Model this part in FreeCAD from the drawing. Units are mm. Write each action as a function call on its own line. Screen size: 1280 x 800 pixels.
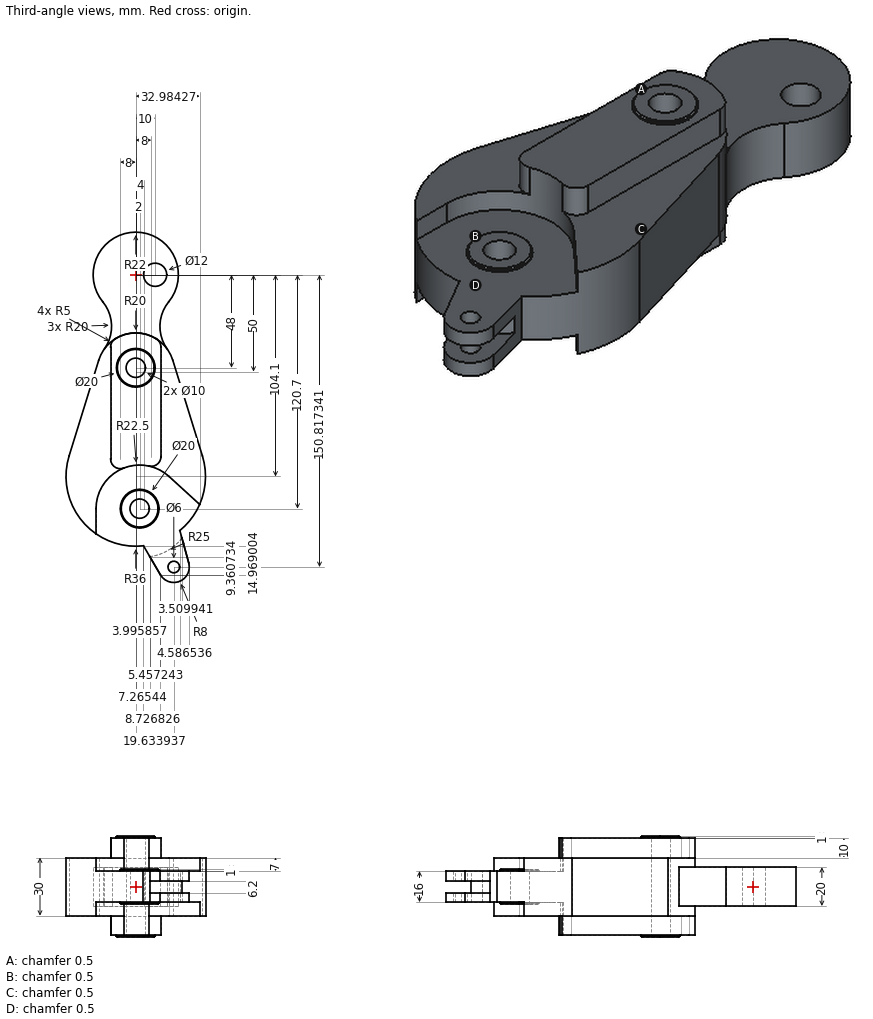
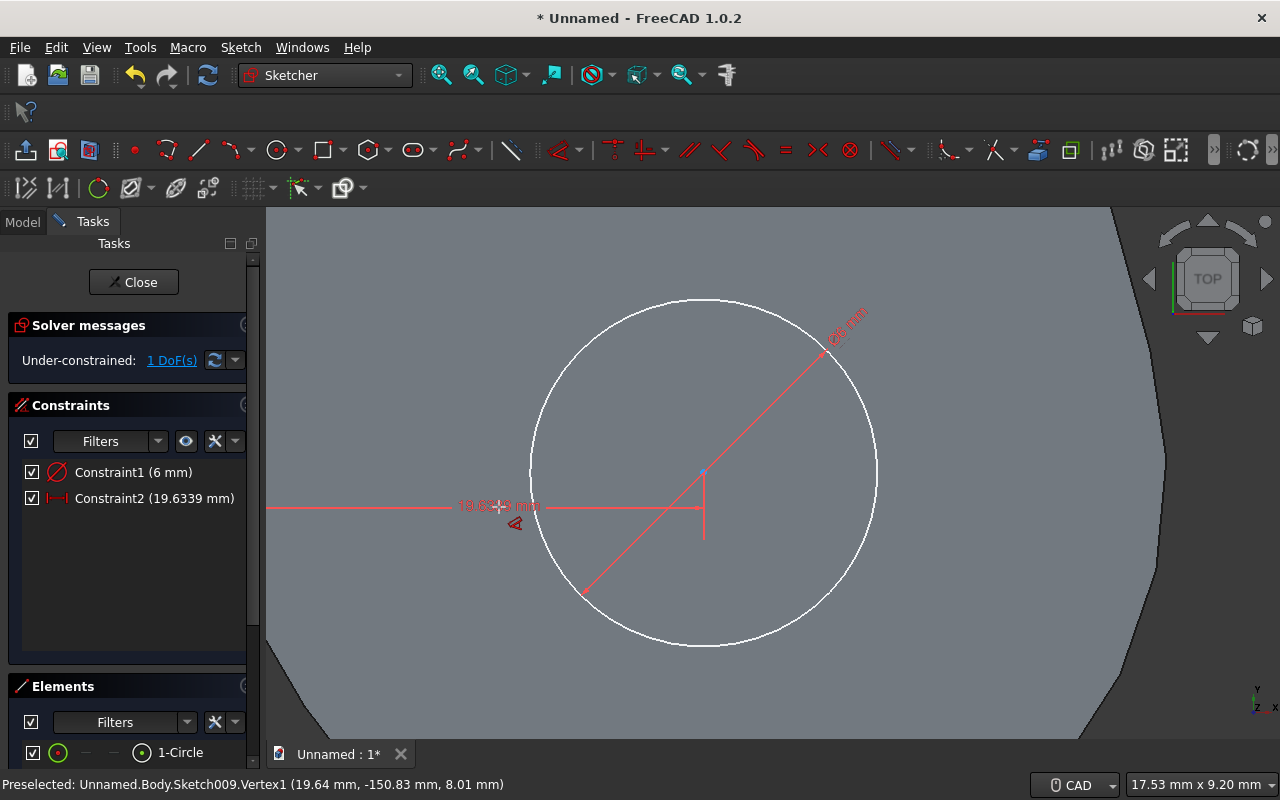
click(704, 473)
click(738, 354)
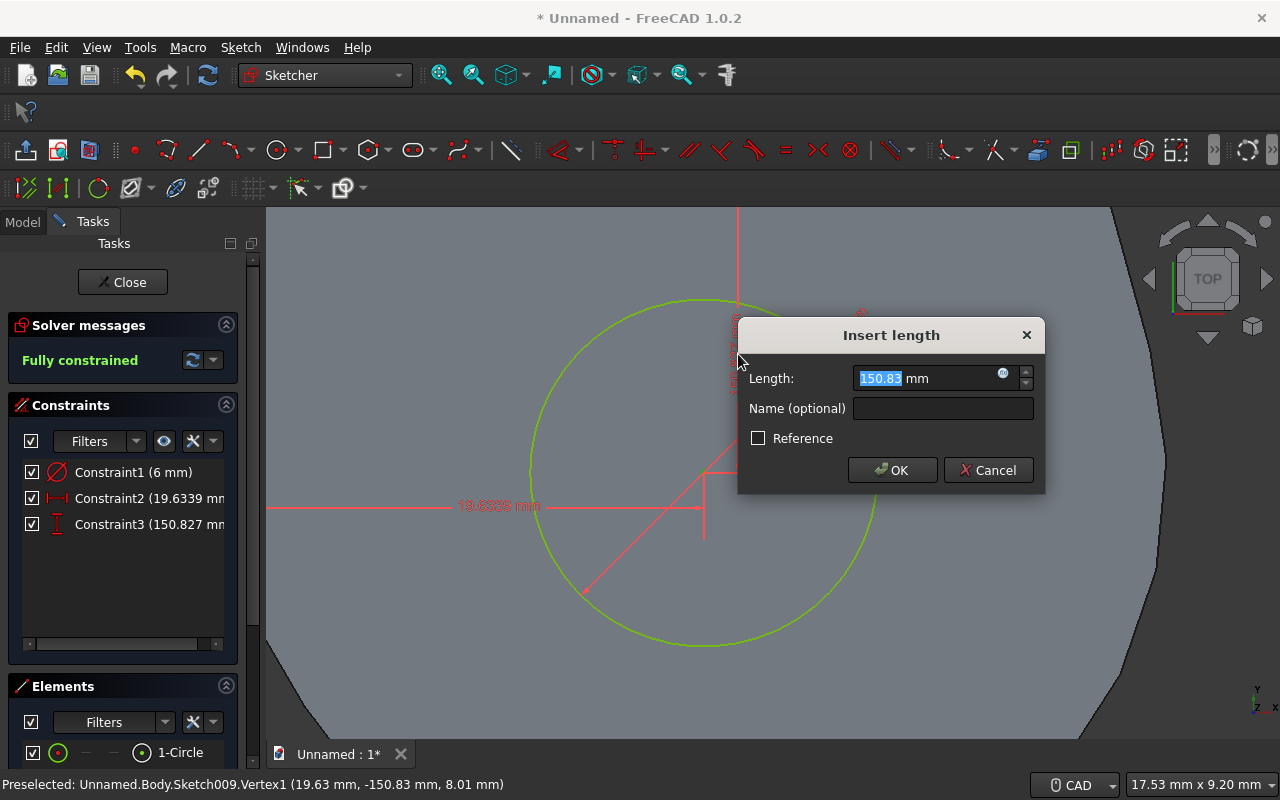
text(150.817341)
key(Return)
key(Escape)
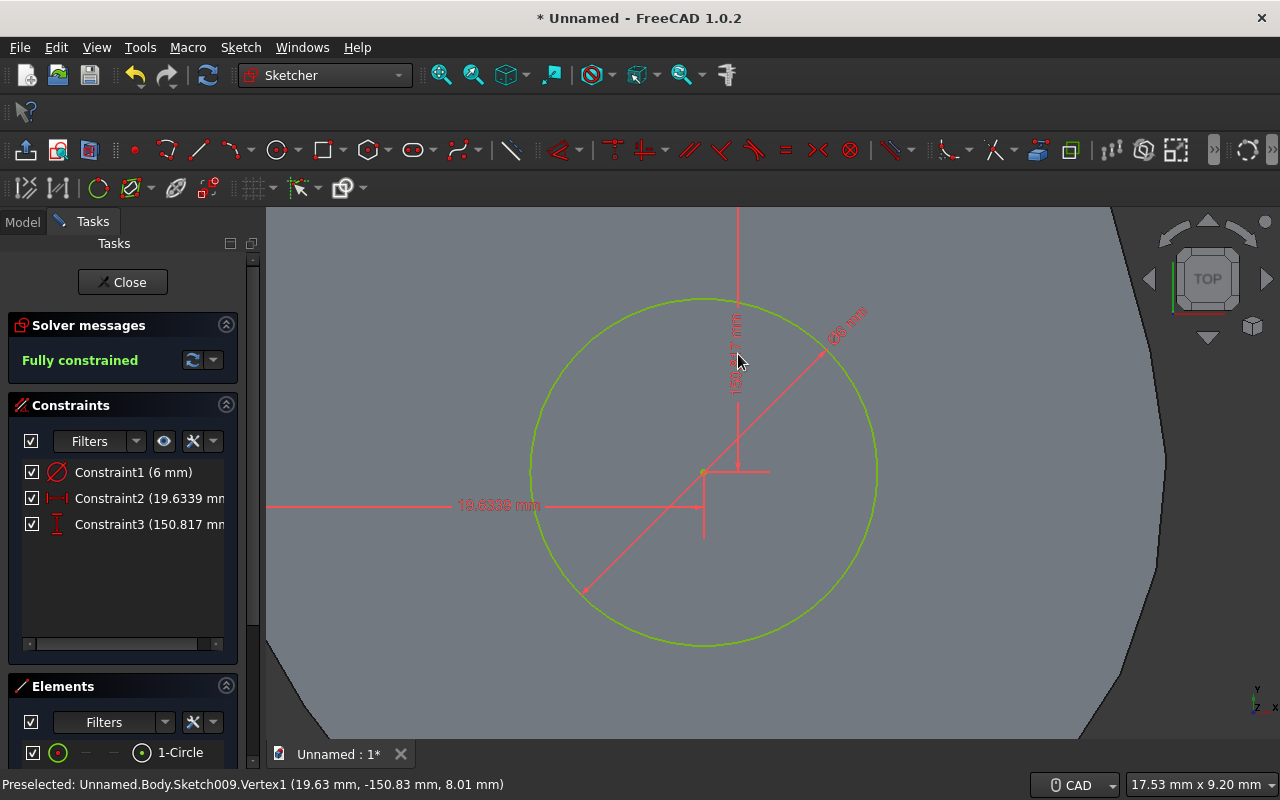
click(123, 282)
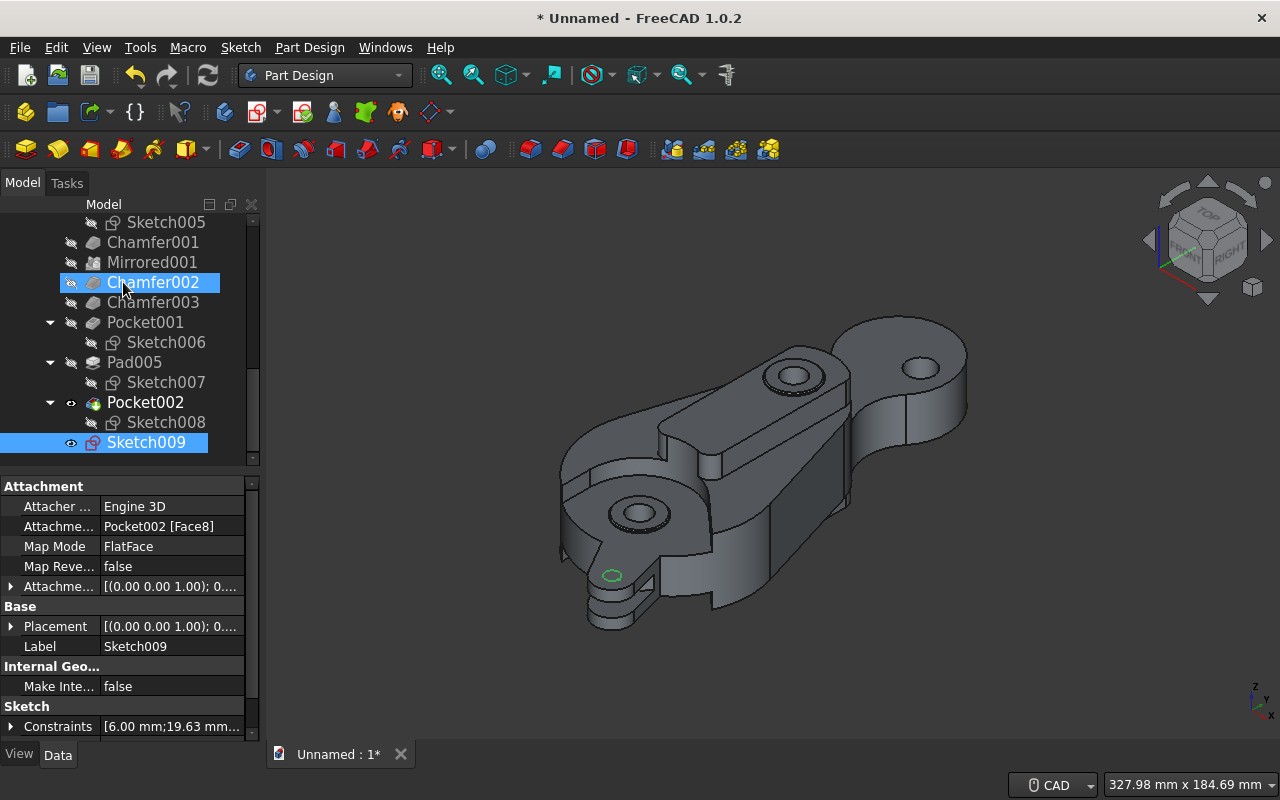
click(240, 150)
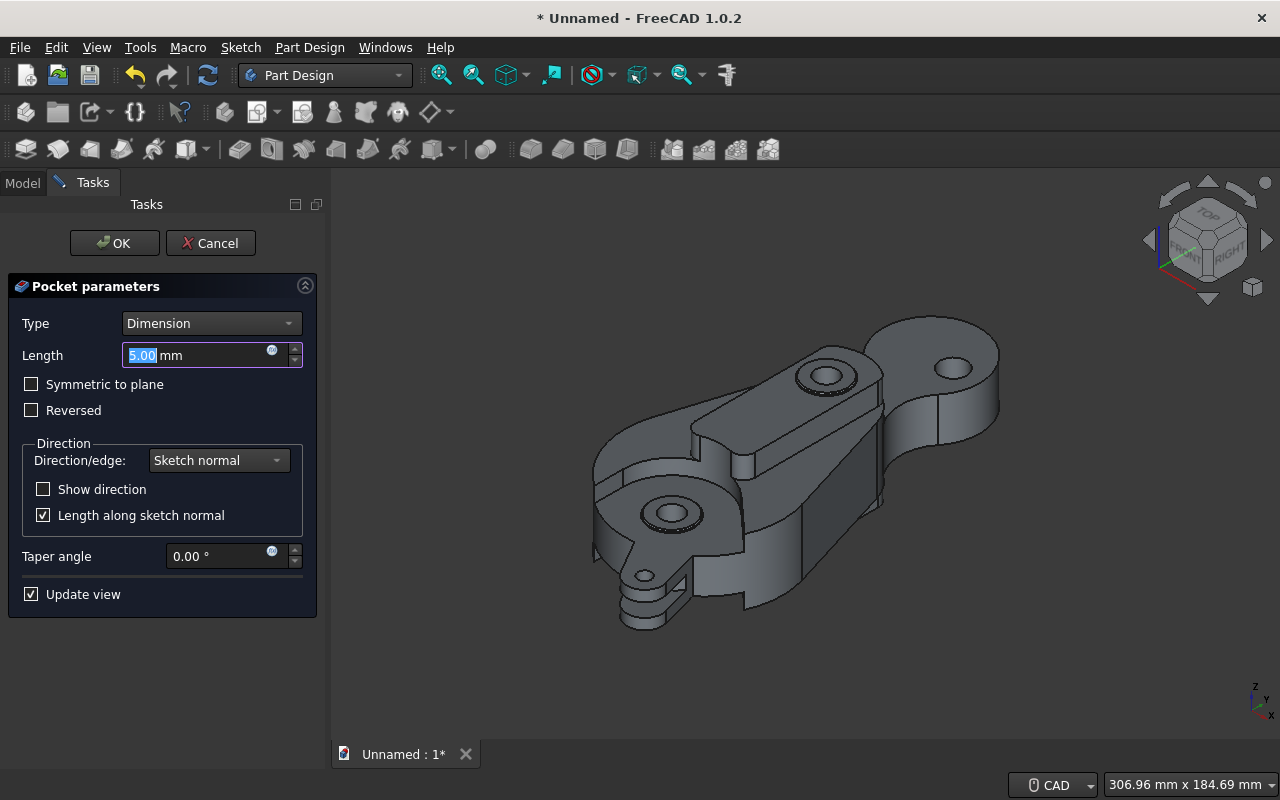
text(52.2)
key(Tab)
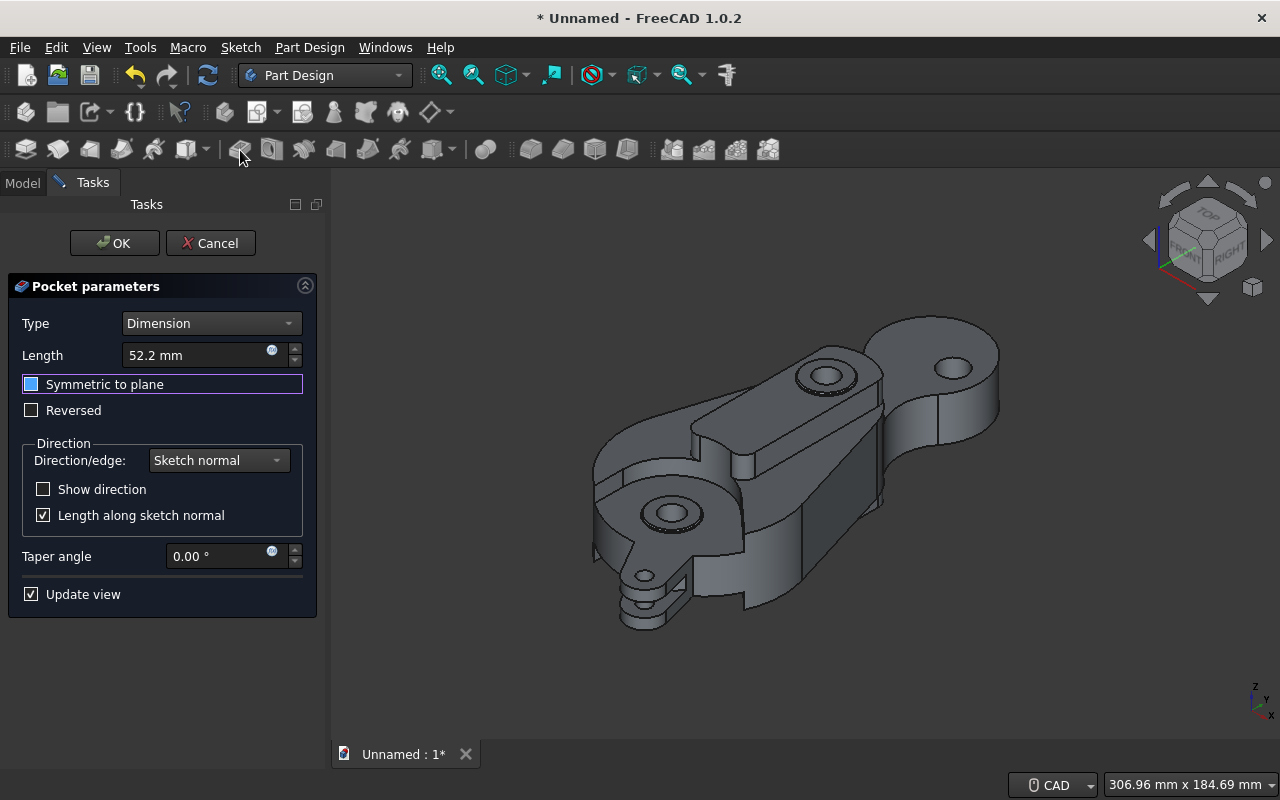
click(30, 384)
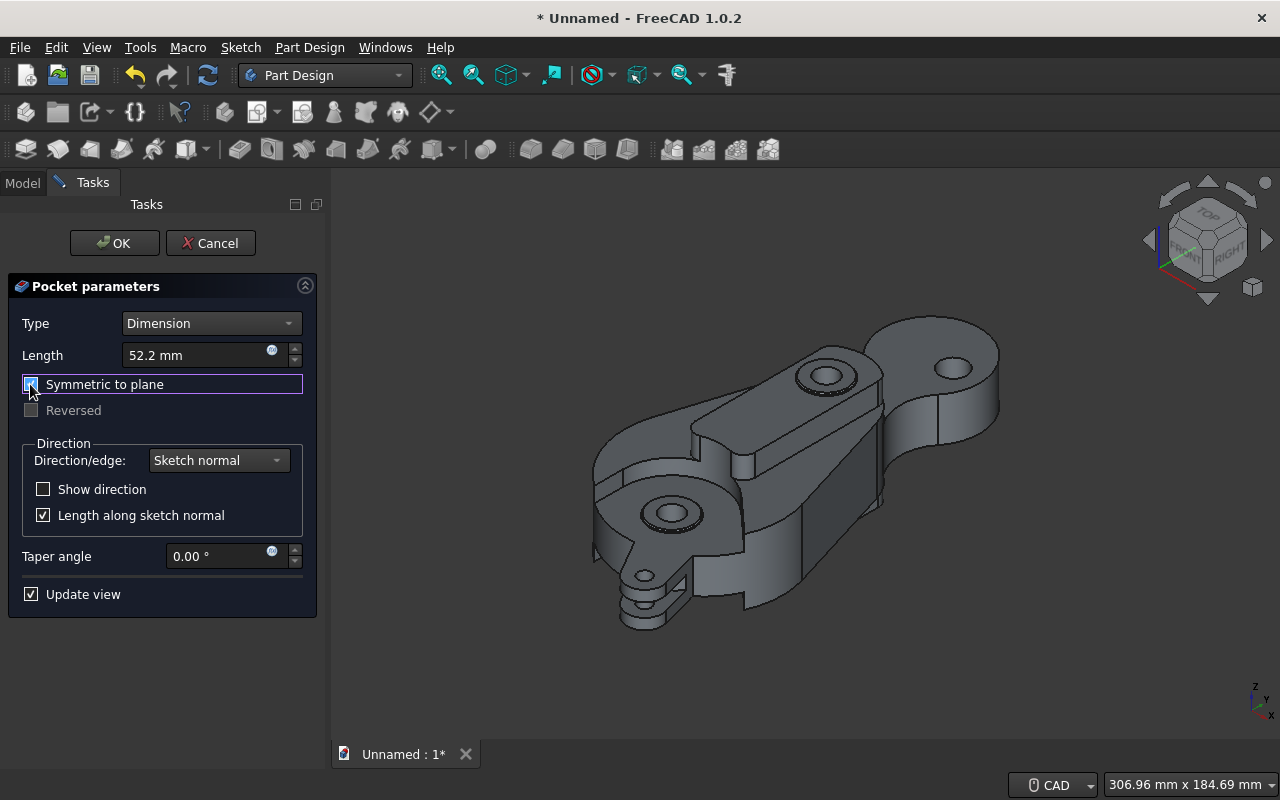
click(115, 243)